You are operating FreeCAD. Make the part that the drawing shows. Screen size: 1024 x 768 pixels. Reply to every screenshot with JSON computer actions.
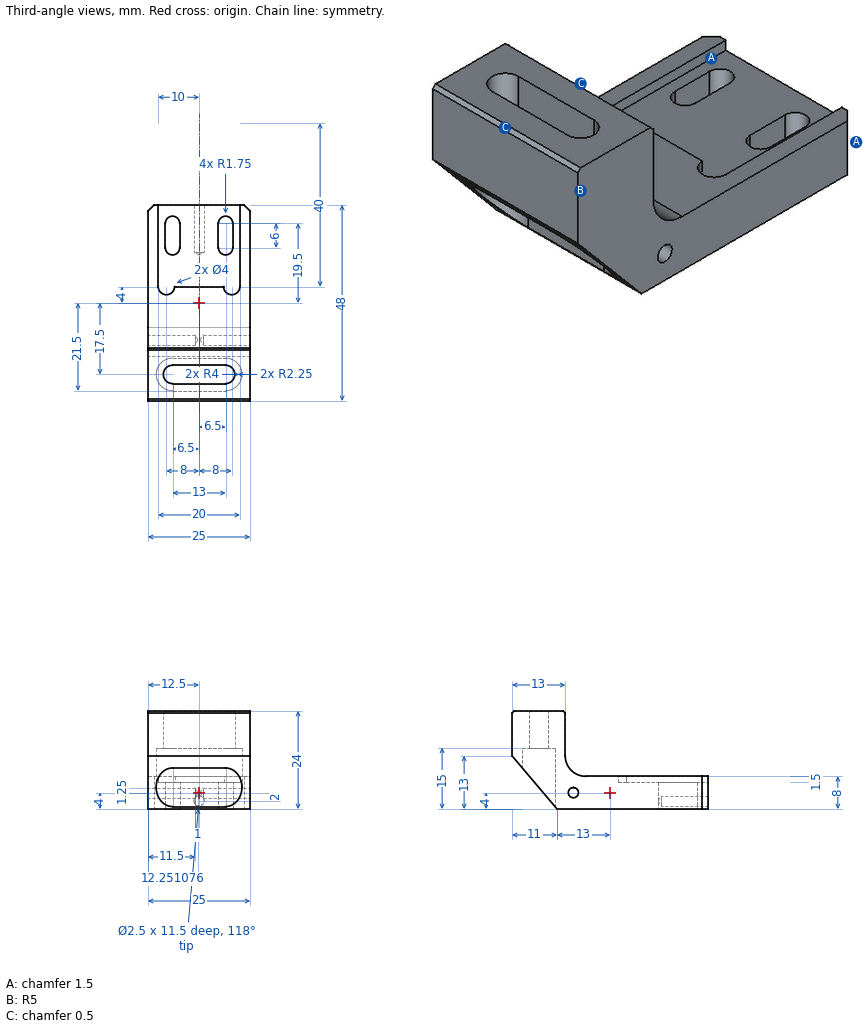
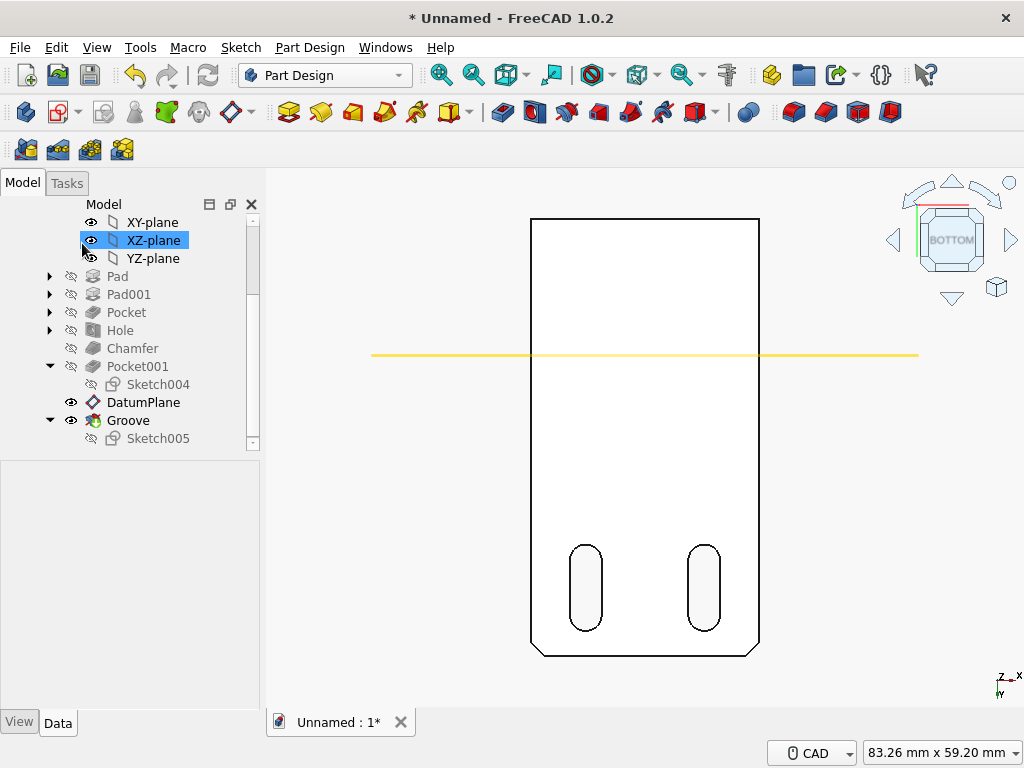
{"action": "left_click", "coordinate": [116, 402]}
{"action": "key", "text": "space"}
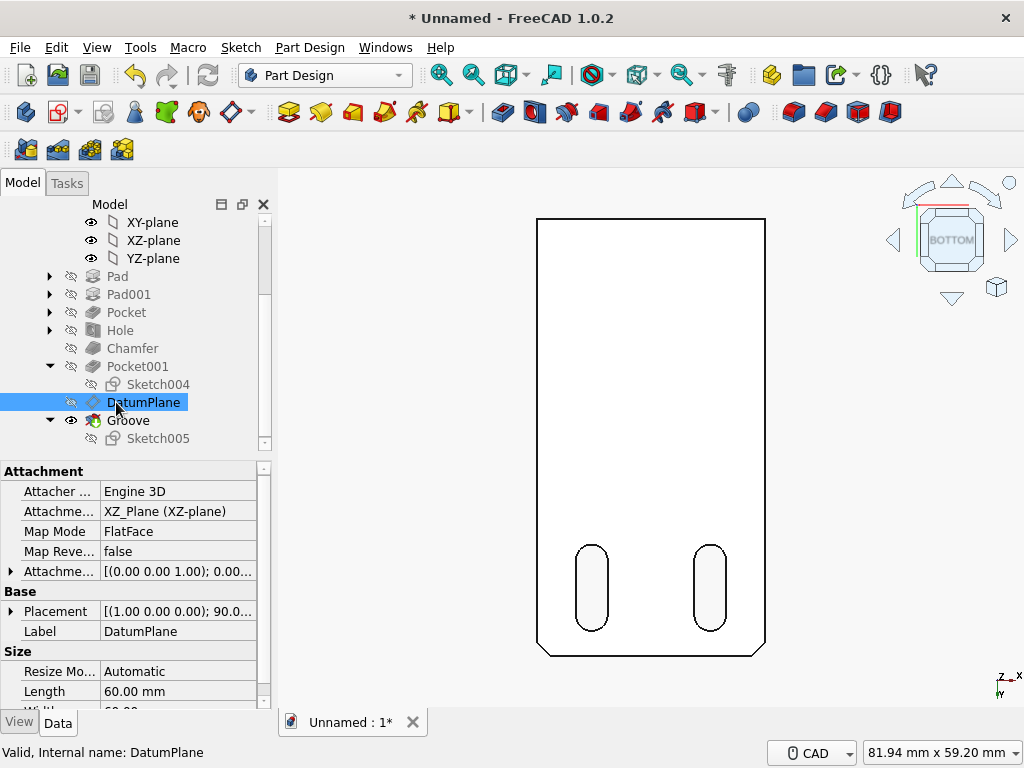
{"action": "key", "text": "0"}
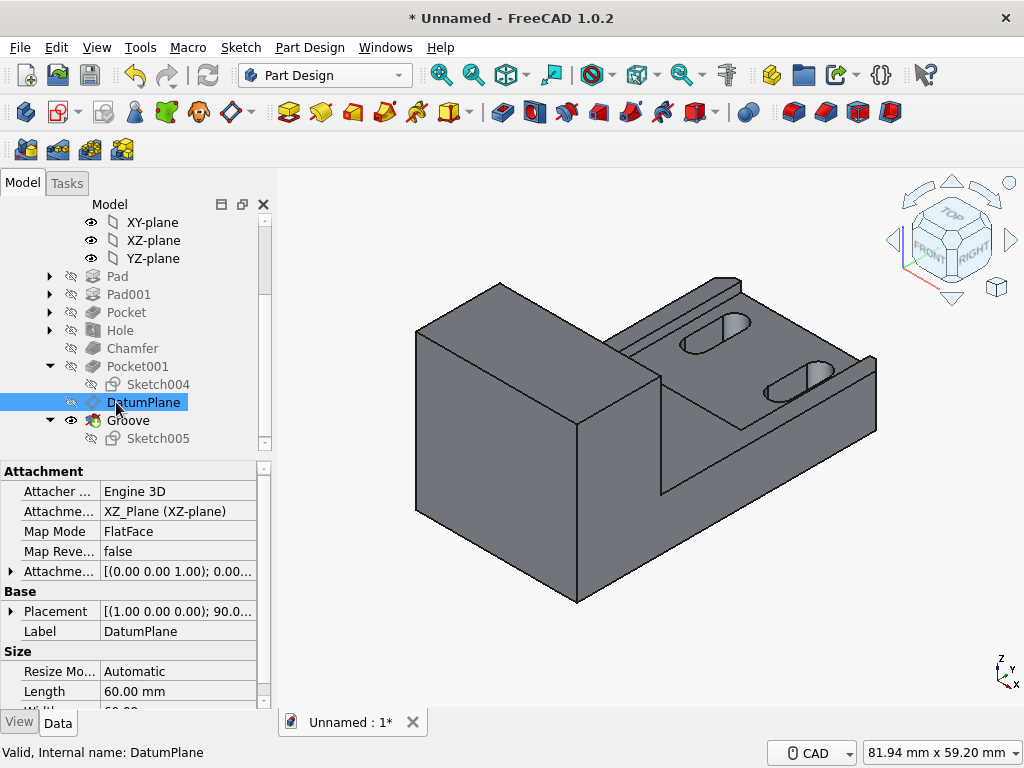
{"action": "left_click", "coordinate": [442, 76]}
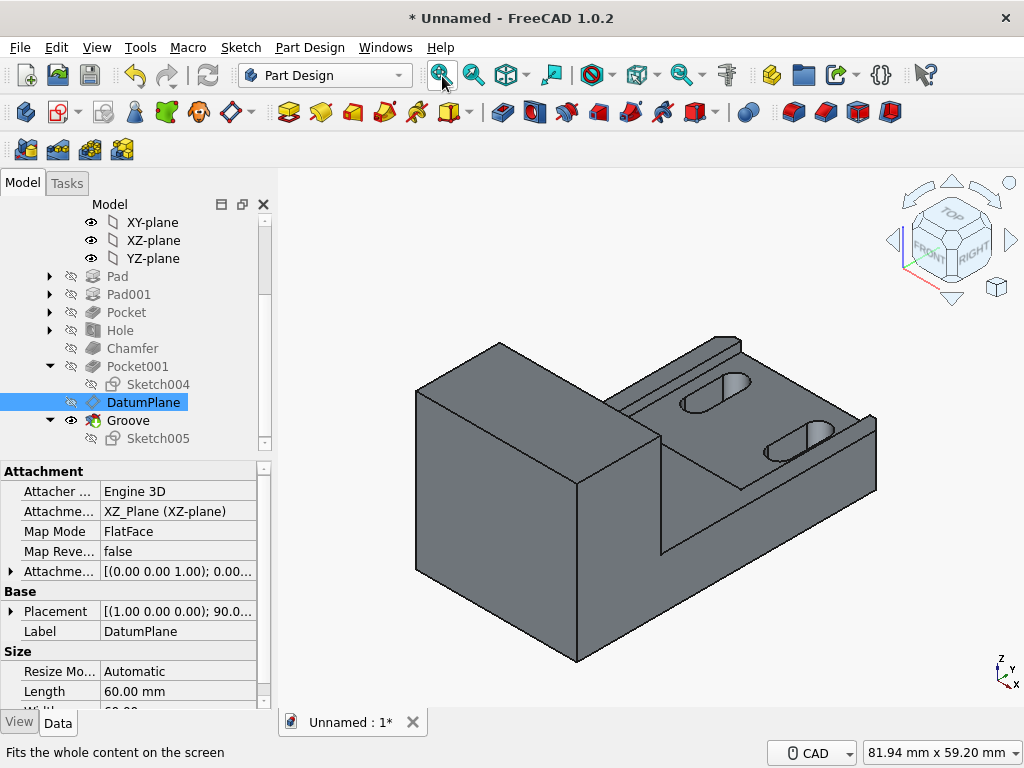
{"action": "left_click", "coordinate": [674, 506]}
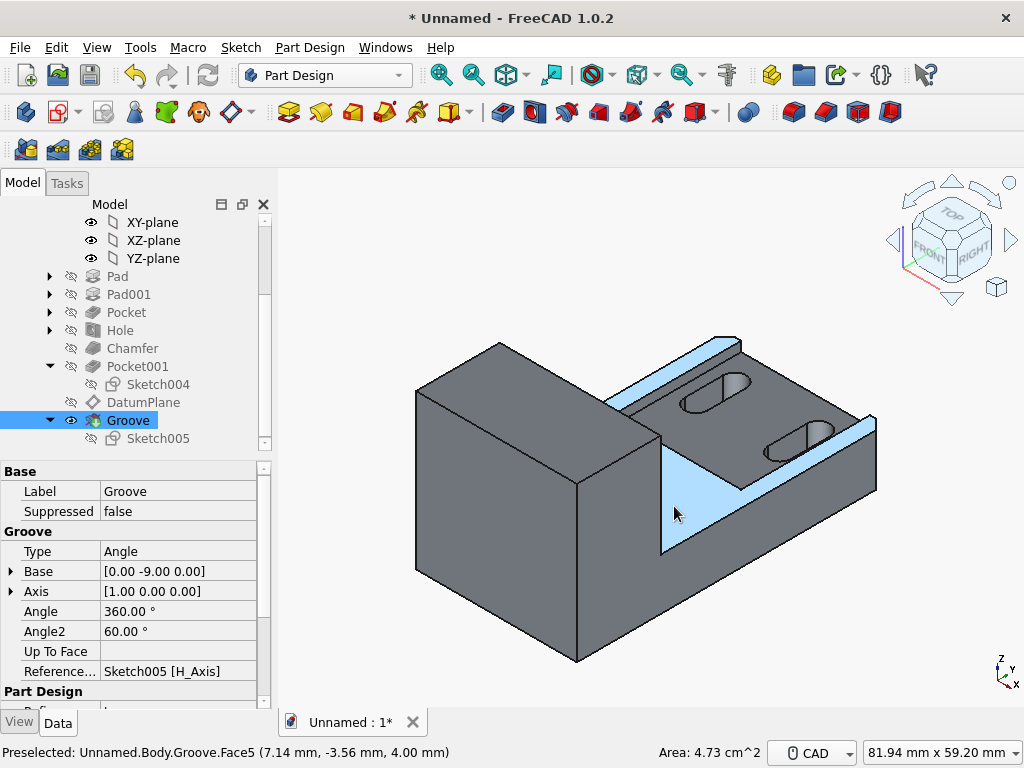
{"action": "left_click", "coordinate": [58, 112]}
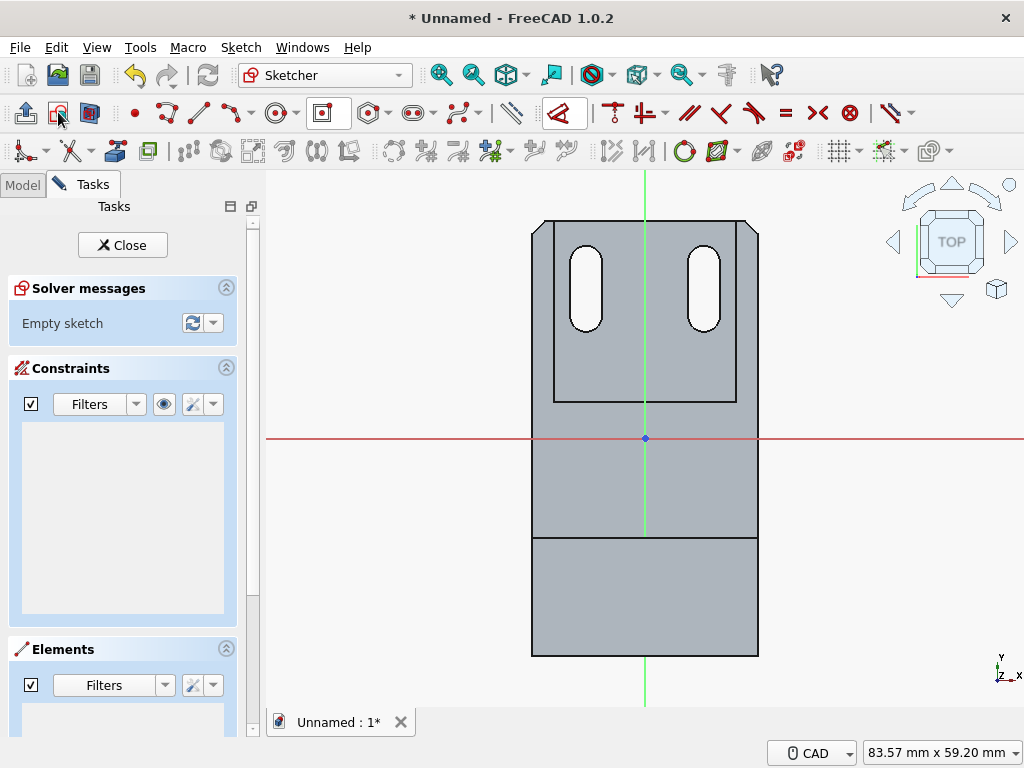
{"action": "left_click", "coordinate": [90, 114]}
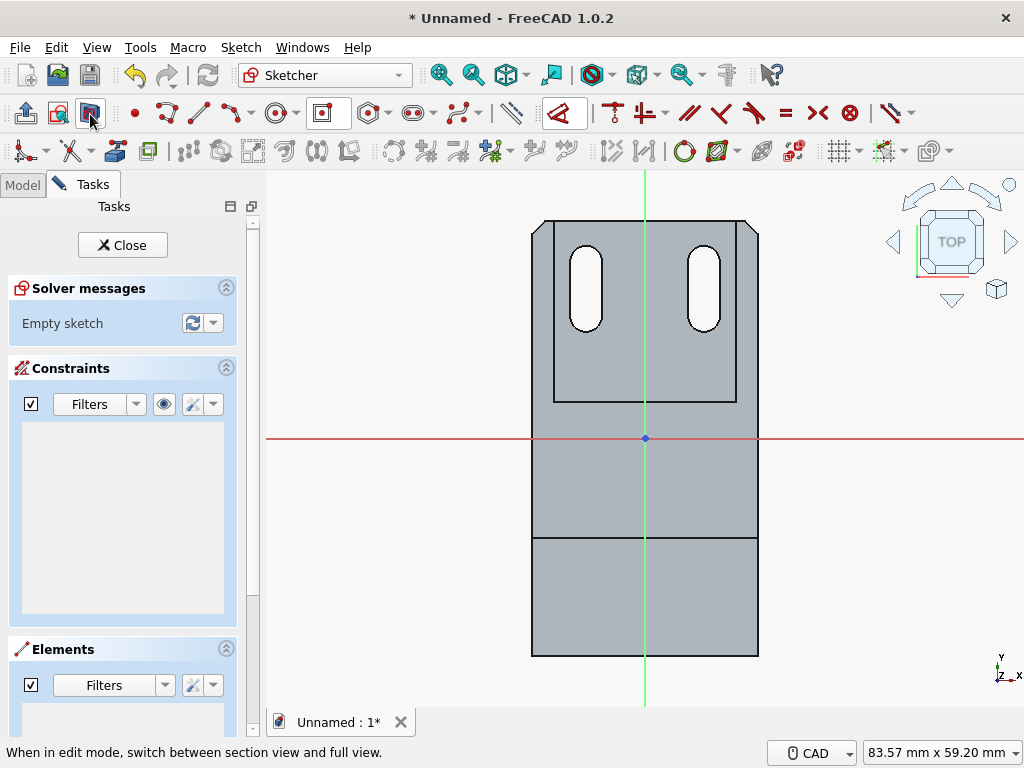
{"action": "scroll", "coordinate": [701, 389], "scroll_direction": "up", "scroll_amount": 4}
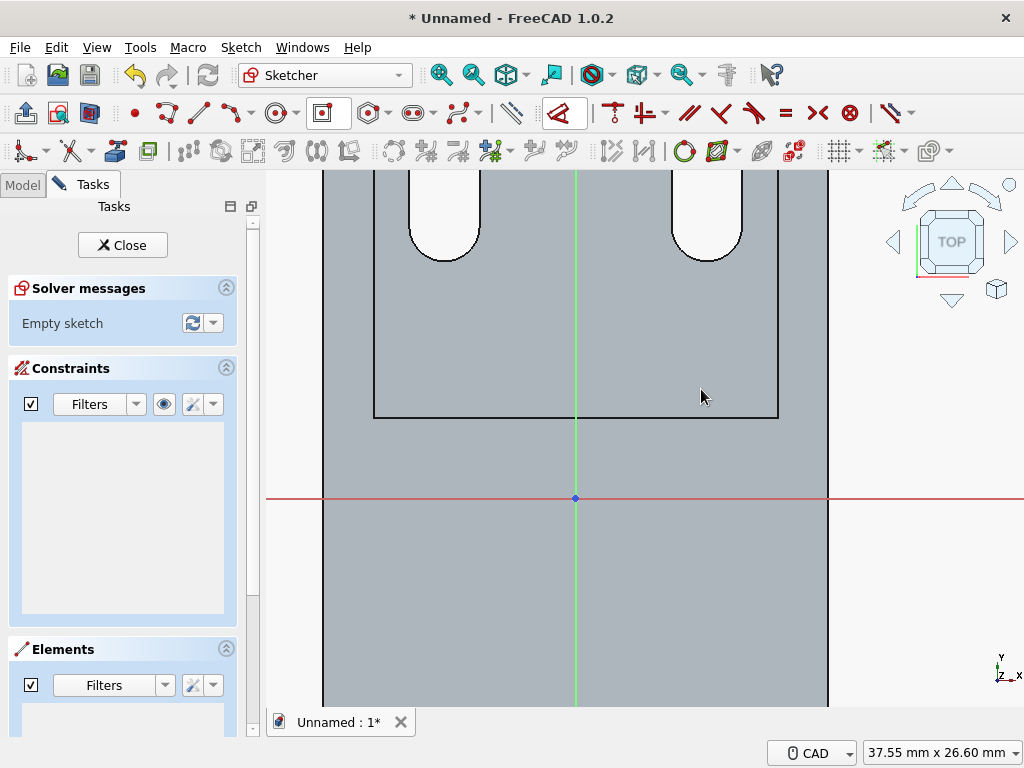
{"action": "left_click", "coordinate": [276, 114]}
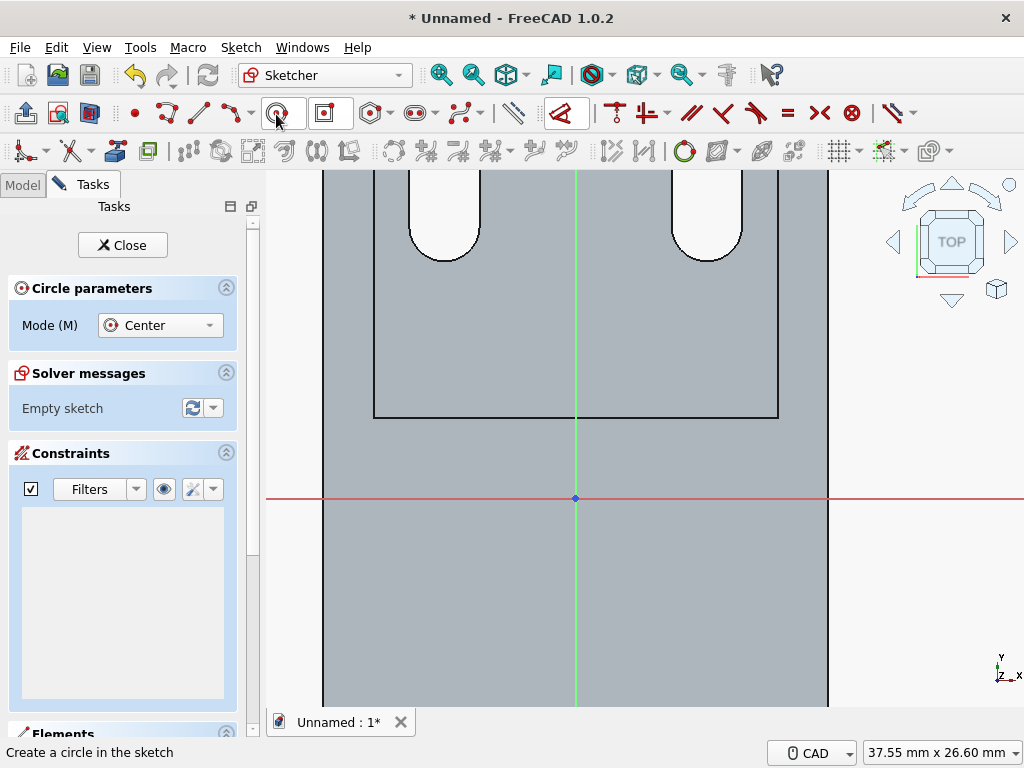
{"action": "left_click", "coordinate": [414, 418]}
{"action": "mouse_move", "coordinate": [443, 389]}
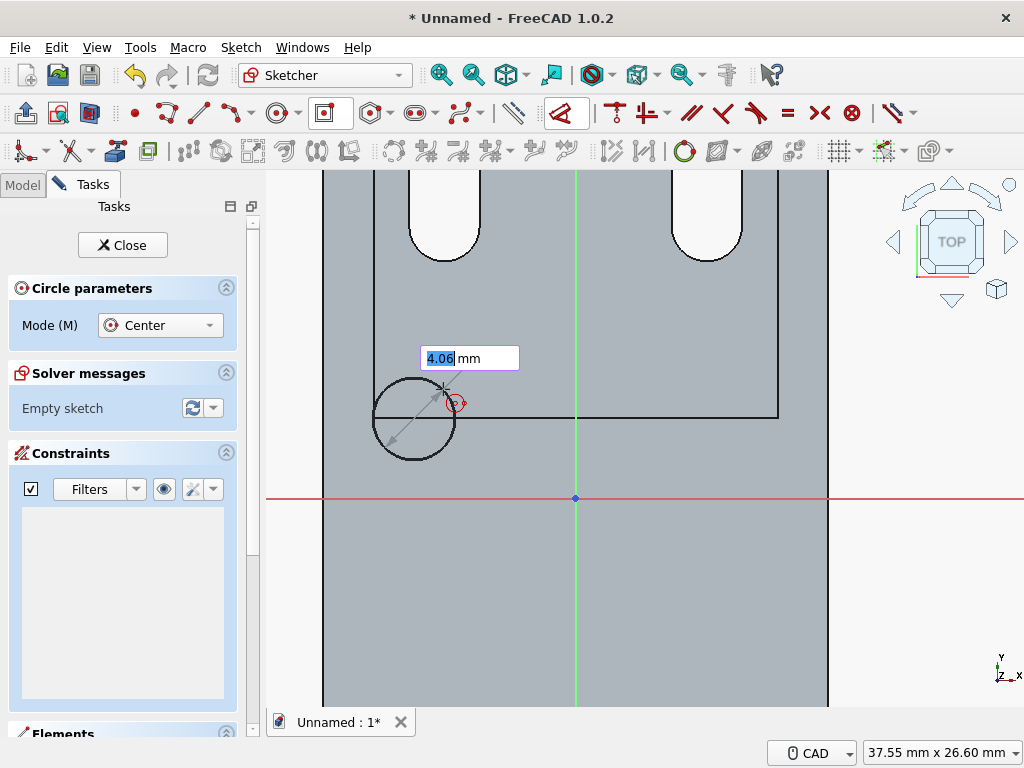
{"action": "type", "text": "4"}
{"action": "key", "text": "Return"}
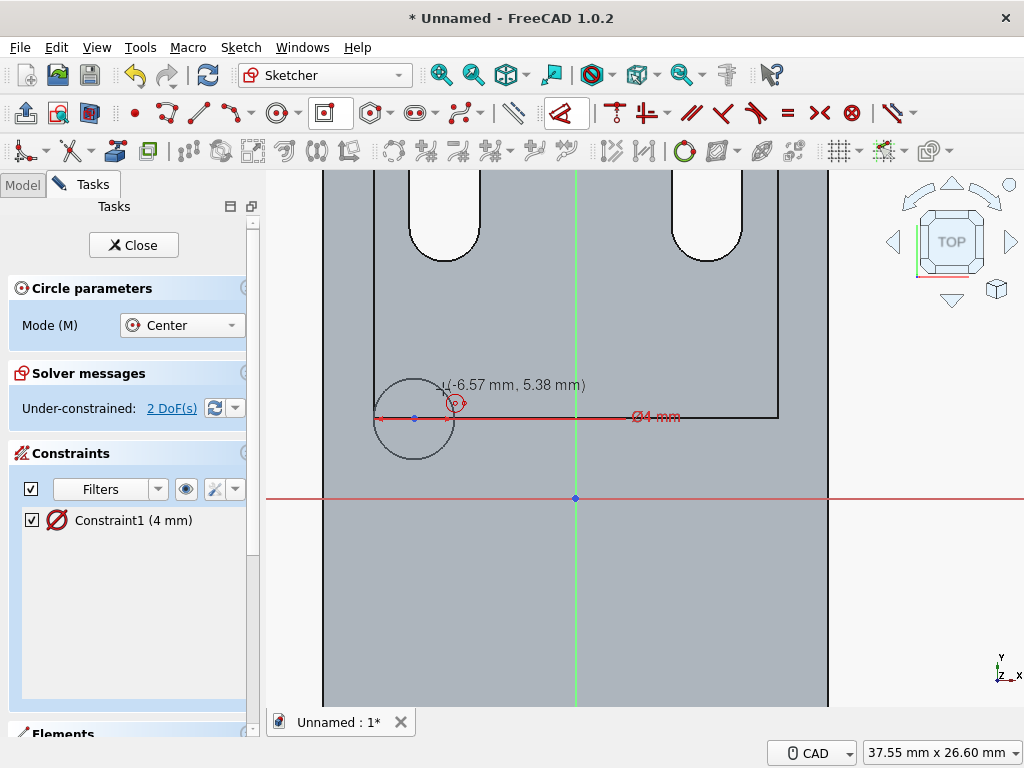
{"action": "left_click", "coordinate": [737, 418]}
{"action": "mouse_move", "coordinate": [766, 389]}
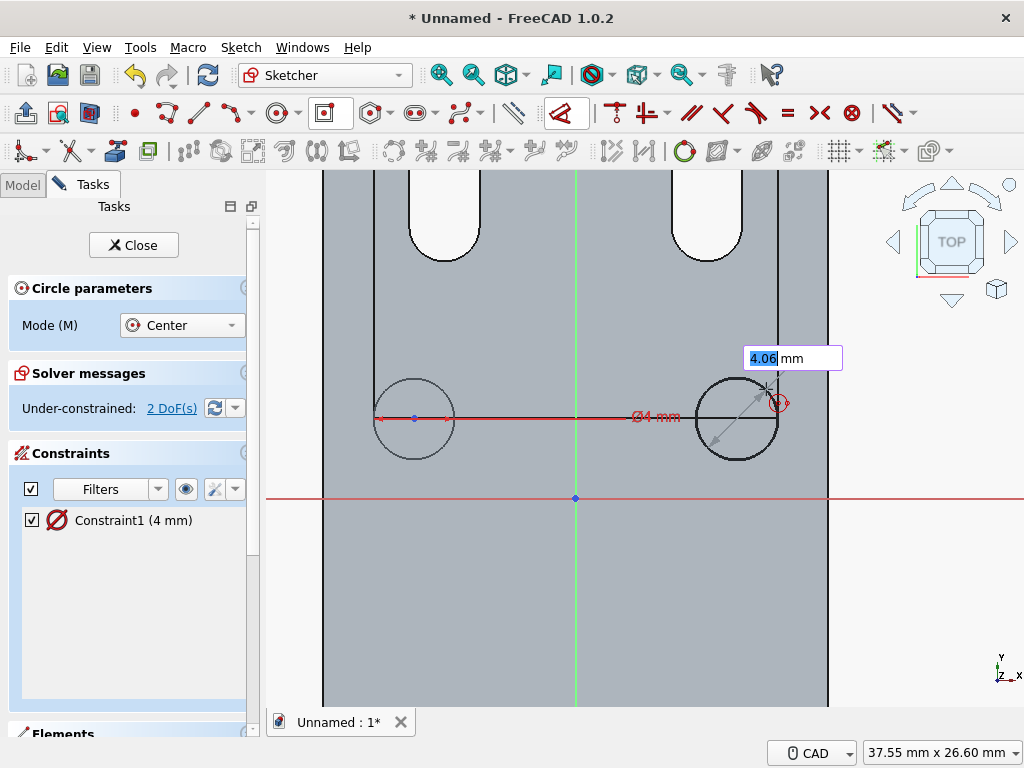
{"action": "type", "text": "4"}
{"action": "key", "text": "Return"}
{"action": "key", "text": "Escape"}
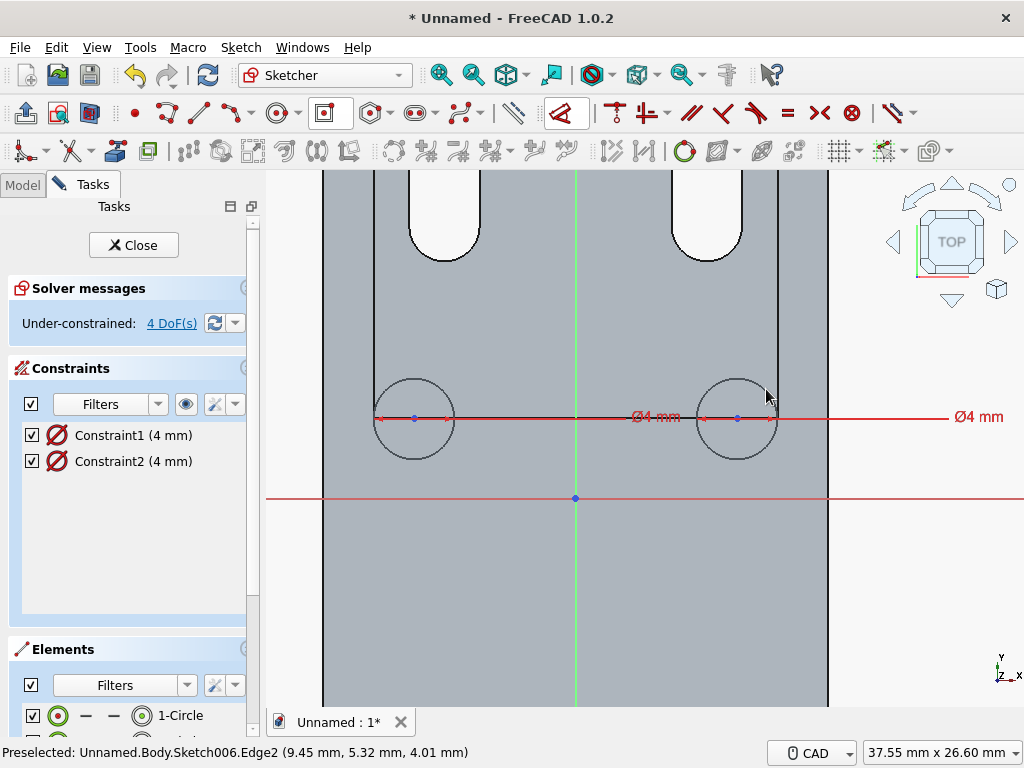
{"action": "left_click", "coordinate": [414, 419]}